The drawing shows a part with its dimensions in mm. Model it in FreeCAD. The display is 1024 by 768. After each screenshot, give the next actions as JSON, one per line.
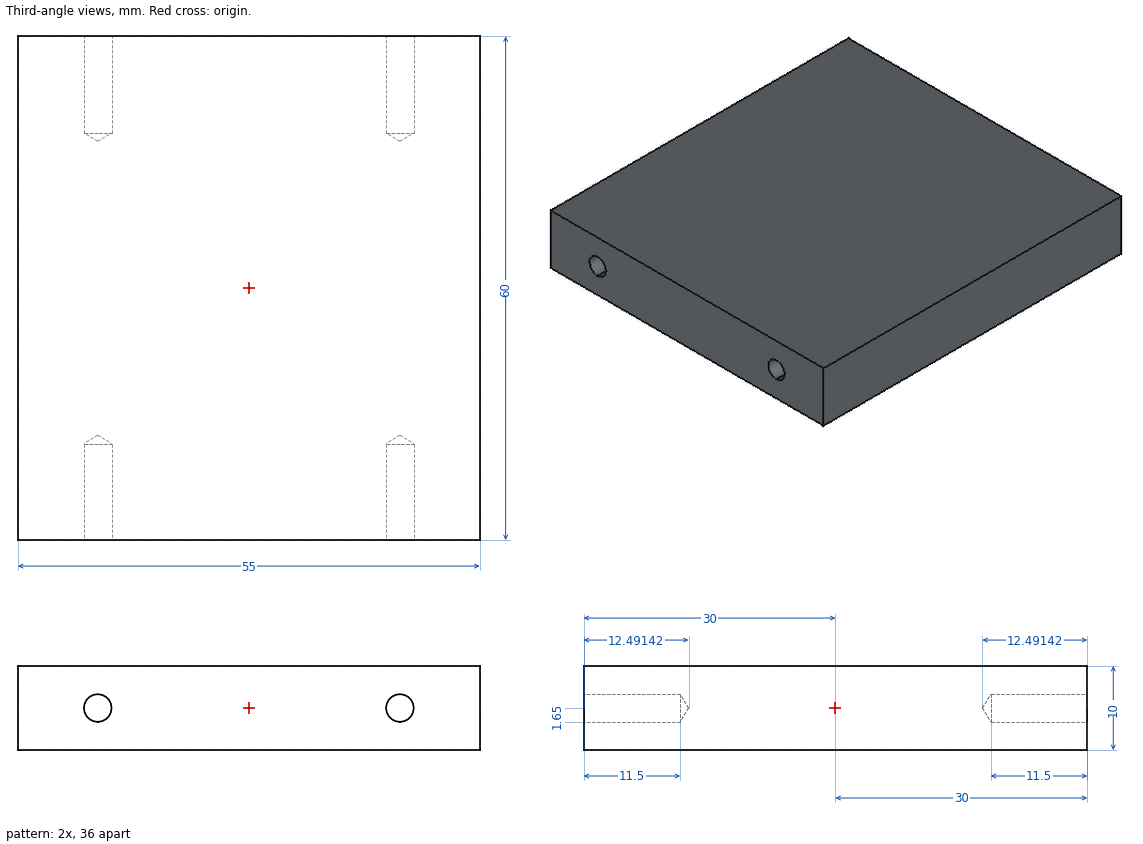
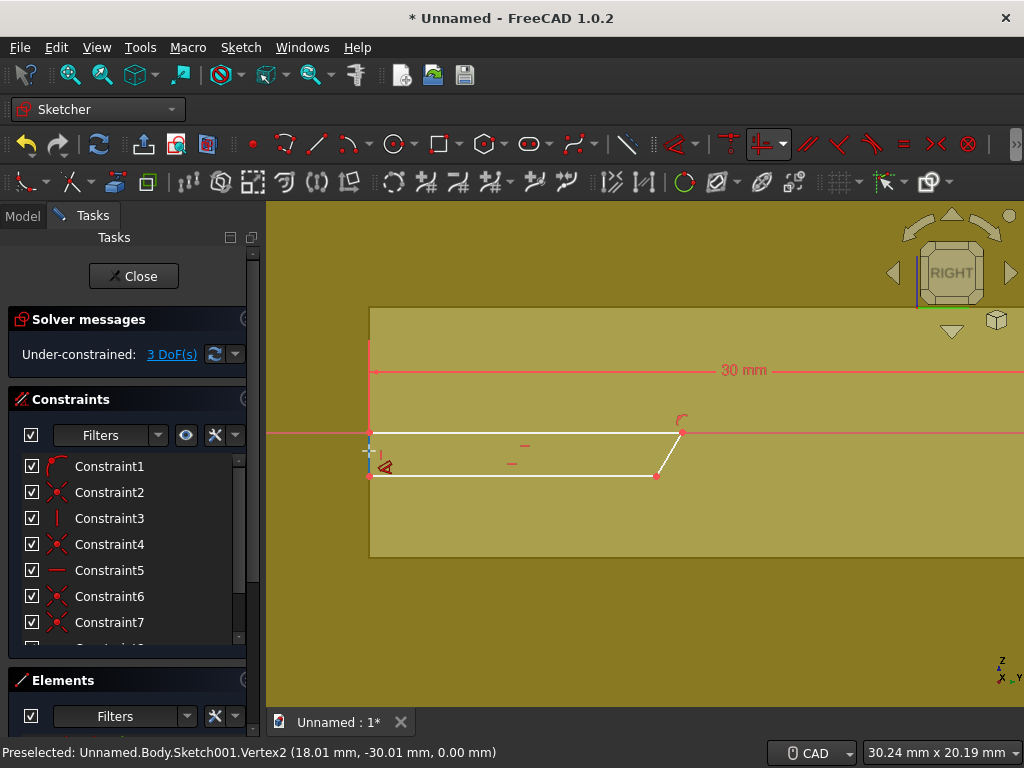
{"action": "left_click", "coordinate": [369, 450]}
{"action": "left_click", "coordinate": [335, 454]}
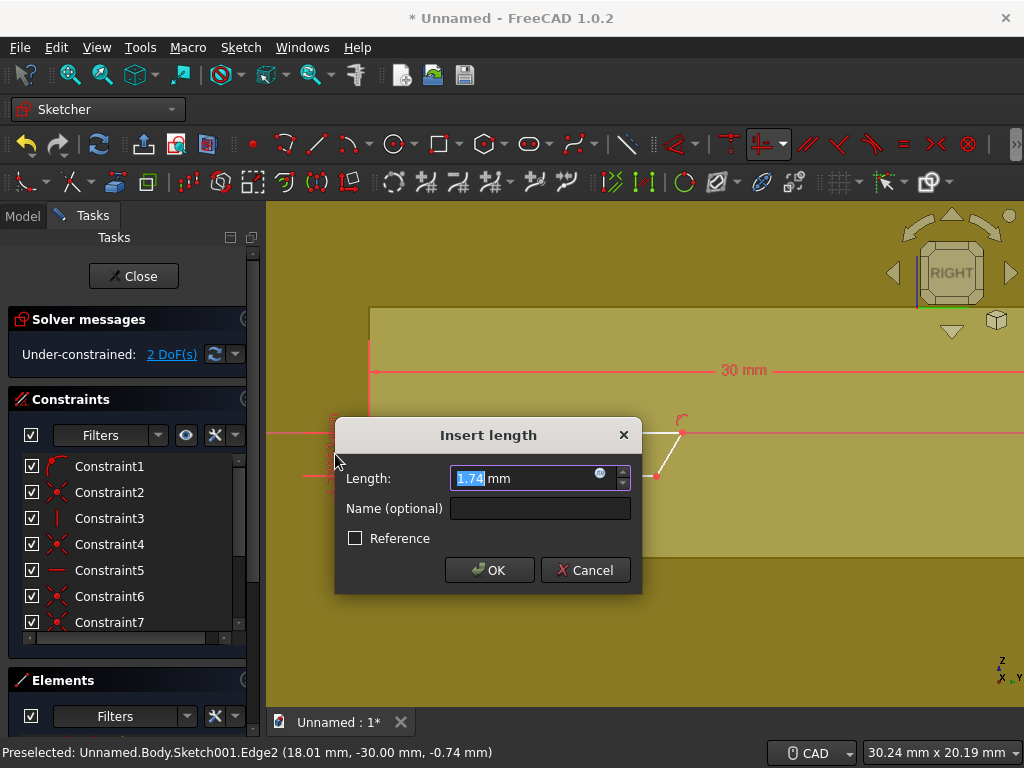
{"action": "type", "text": "1.65"}
{"action": "key", "text": "Return"}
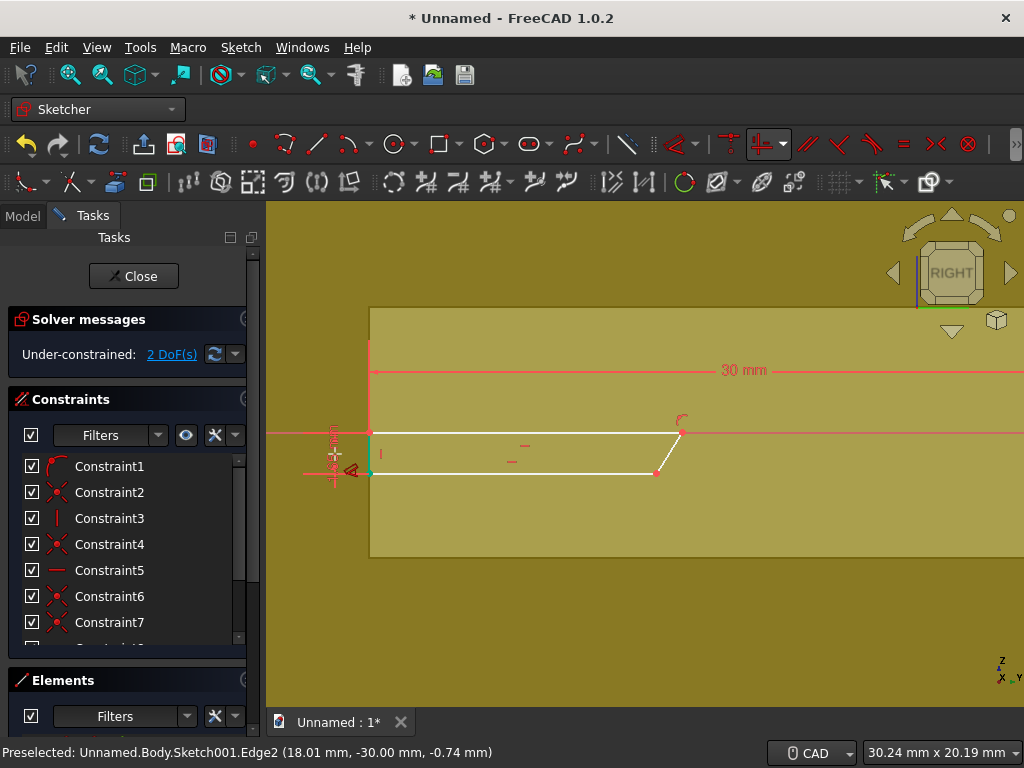
{"action": "left_click", "coordinate": [455, 474]}
{"action": "left_click", "coordinate": [513, 508]}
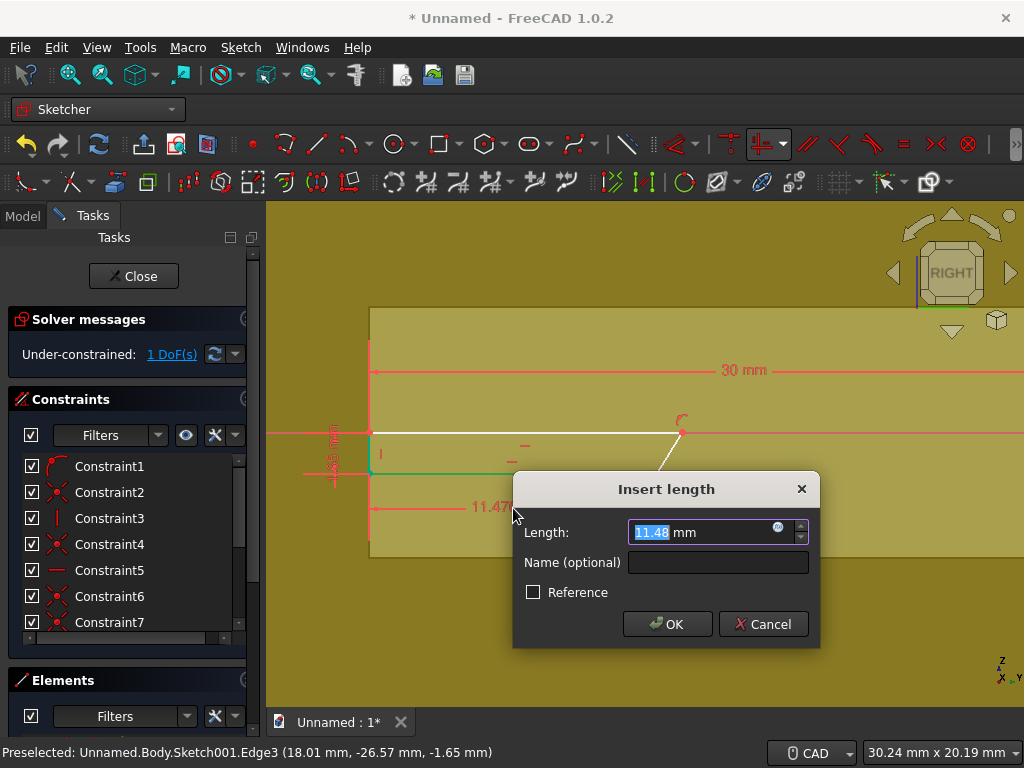
{"action": "type", "text": "11.5"}
{"action": "key", "text": "Return"}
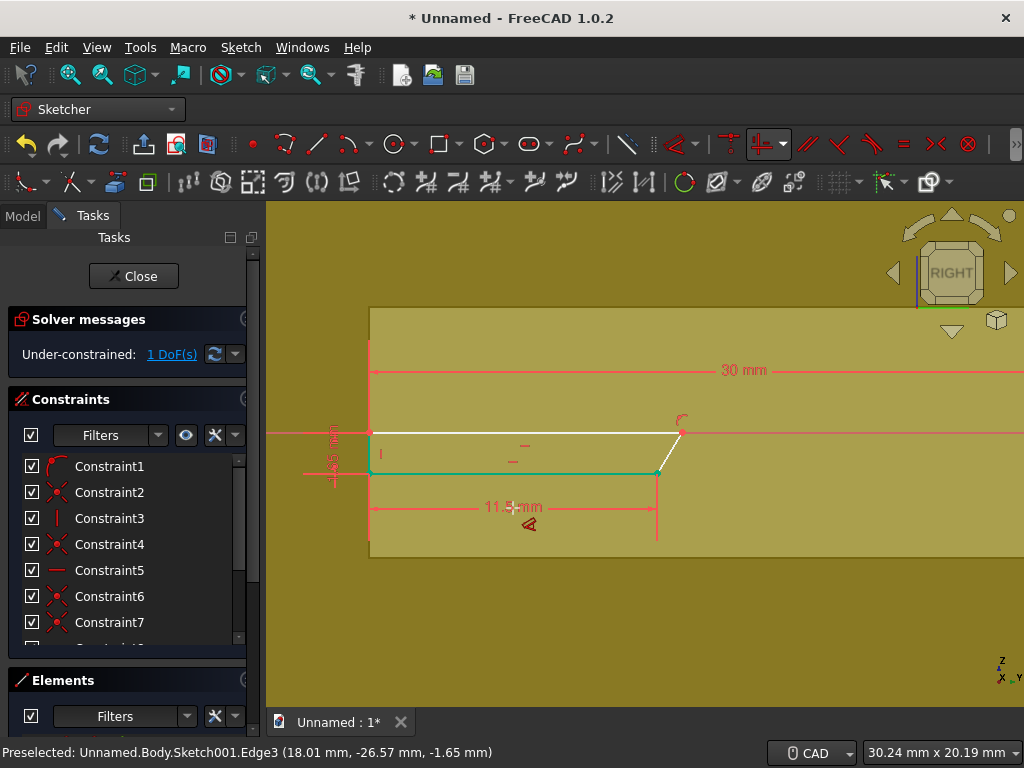
{"action": "left_click", "coordinate": [588, 433]}
{"action": "left_click", "coordinate": [526, 399]}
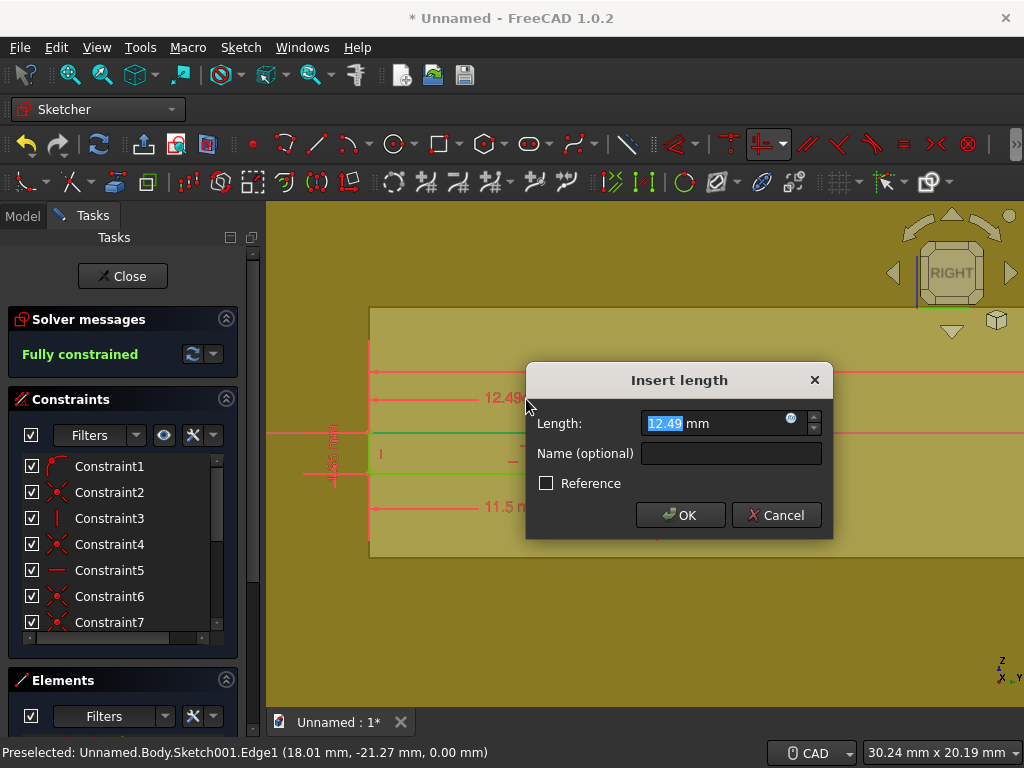
{"action": "type", "text": "12.49142"}
{"action": "key", "text": "Return"}
{"action": "key", "text": "Escape"}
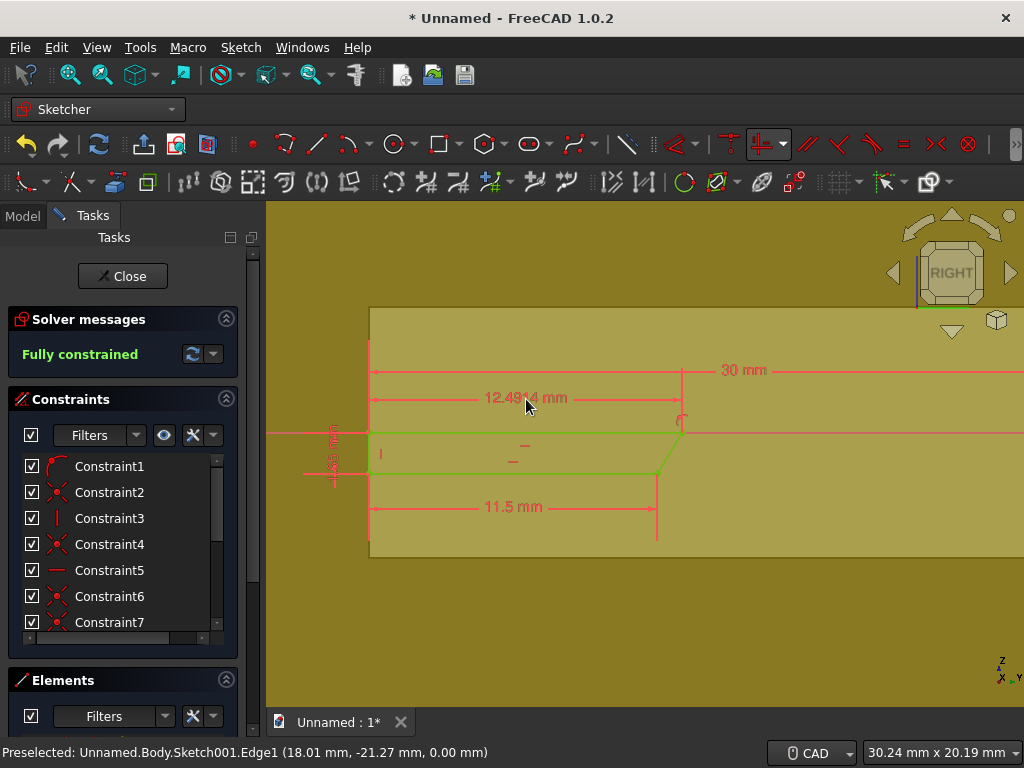
{"action": "left_click", "coordinate": [123, 276]}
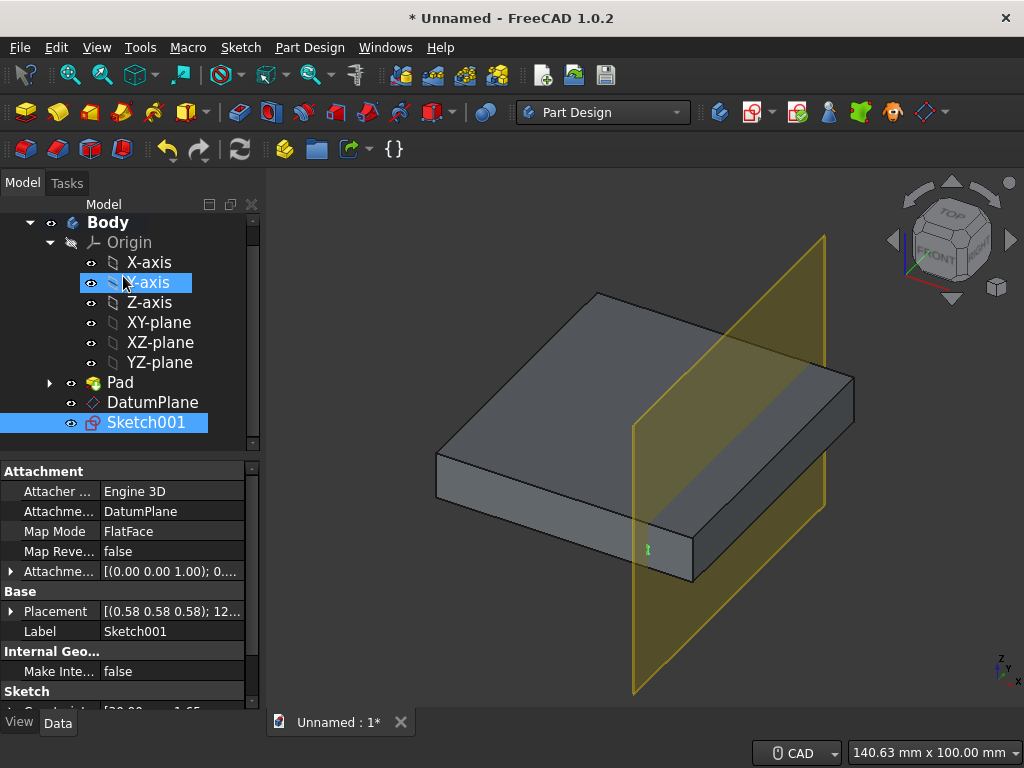
{"action": "left_click", "coordinate": [304, 112]}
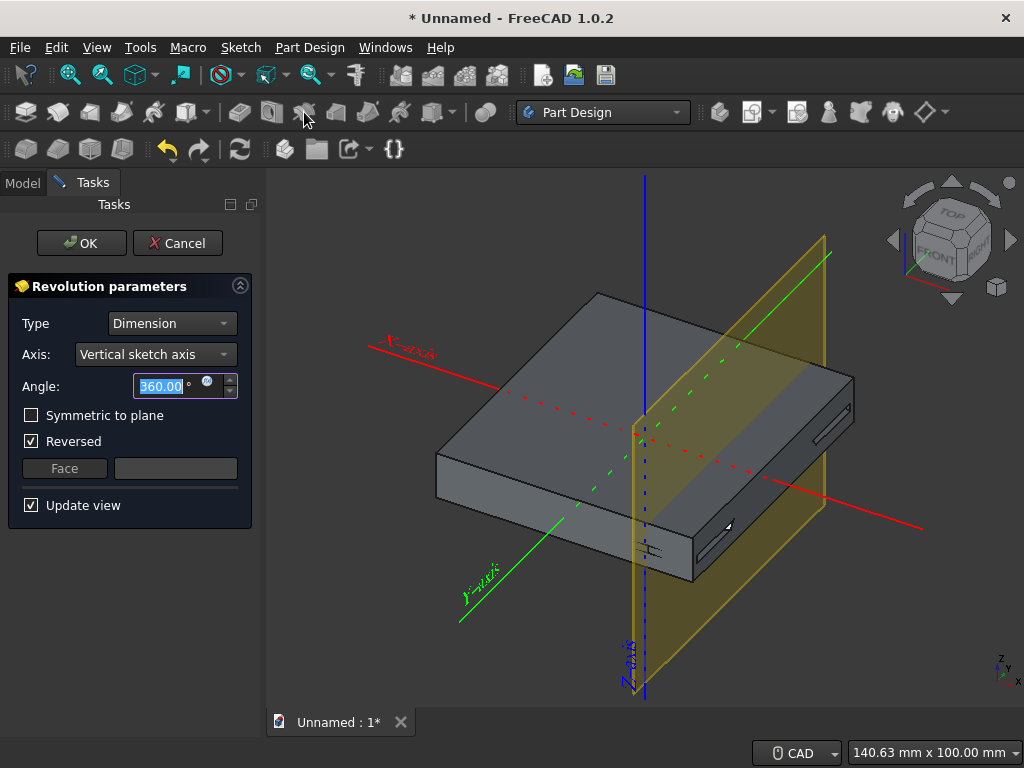
{"action": "left_click", "coordinate": [156, 354]}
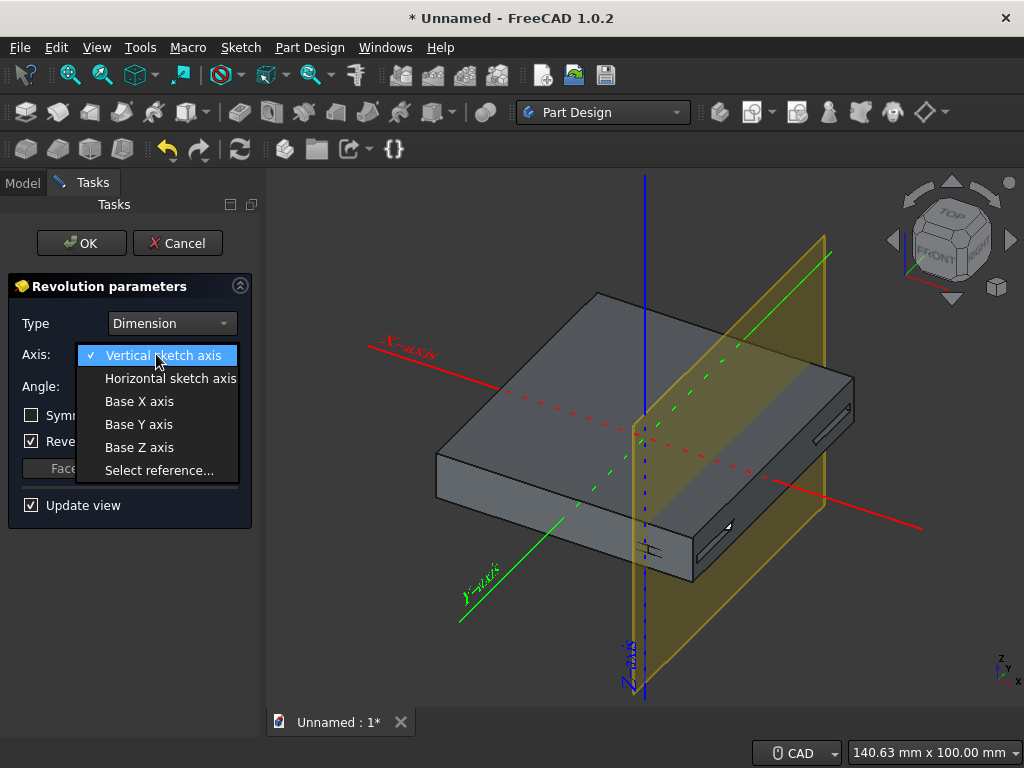
{"action": "left_click", "coordinate": [156, 378]}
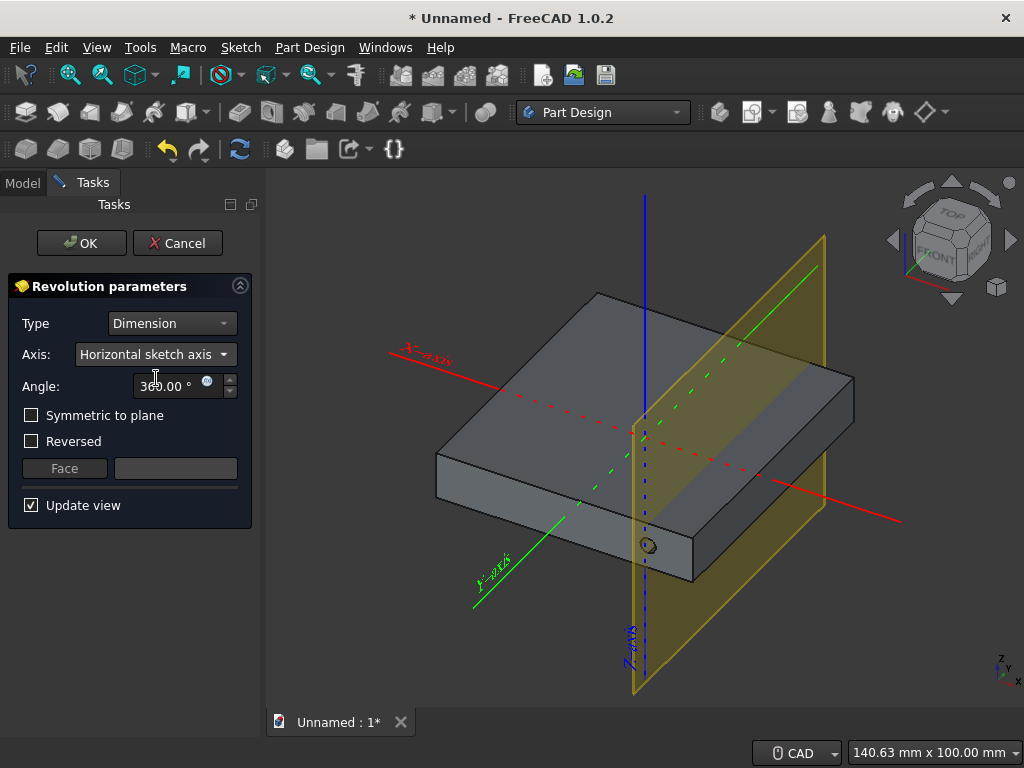
{"action": "left_click", "coordinate": [82, 243]}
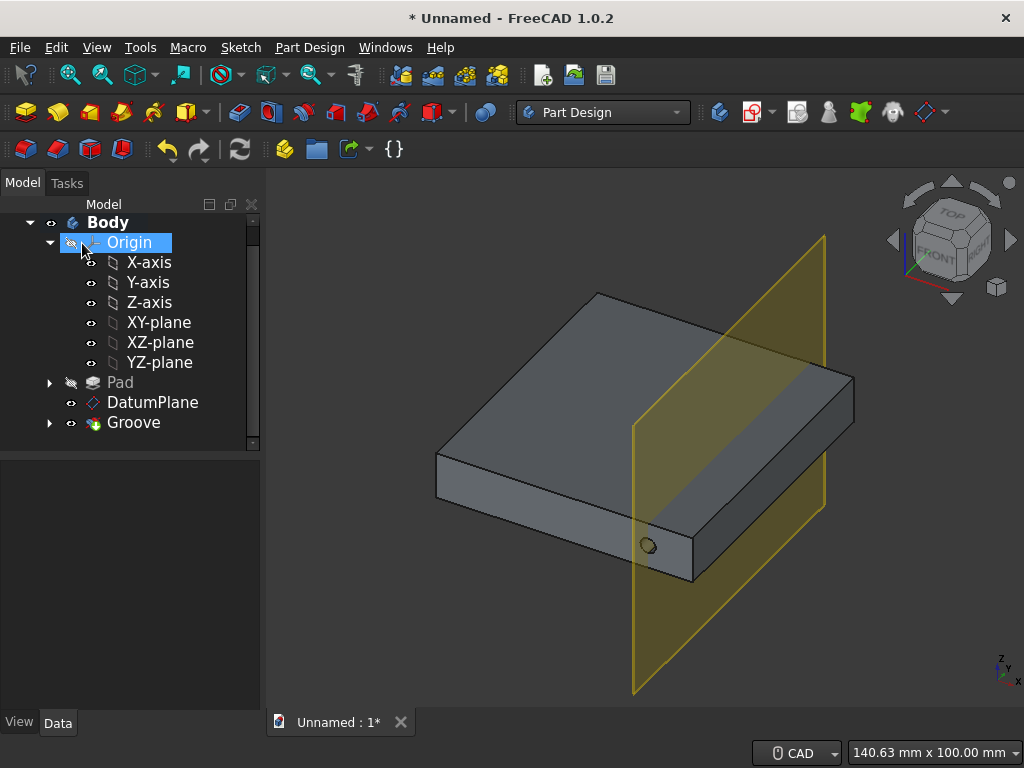
{"action": "left_click", "coordinate": [116, 403]}
{"action": "key", "text": "space"}